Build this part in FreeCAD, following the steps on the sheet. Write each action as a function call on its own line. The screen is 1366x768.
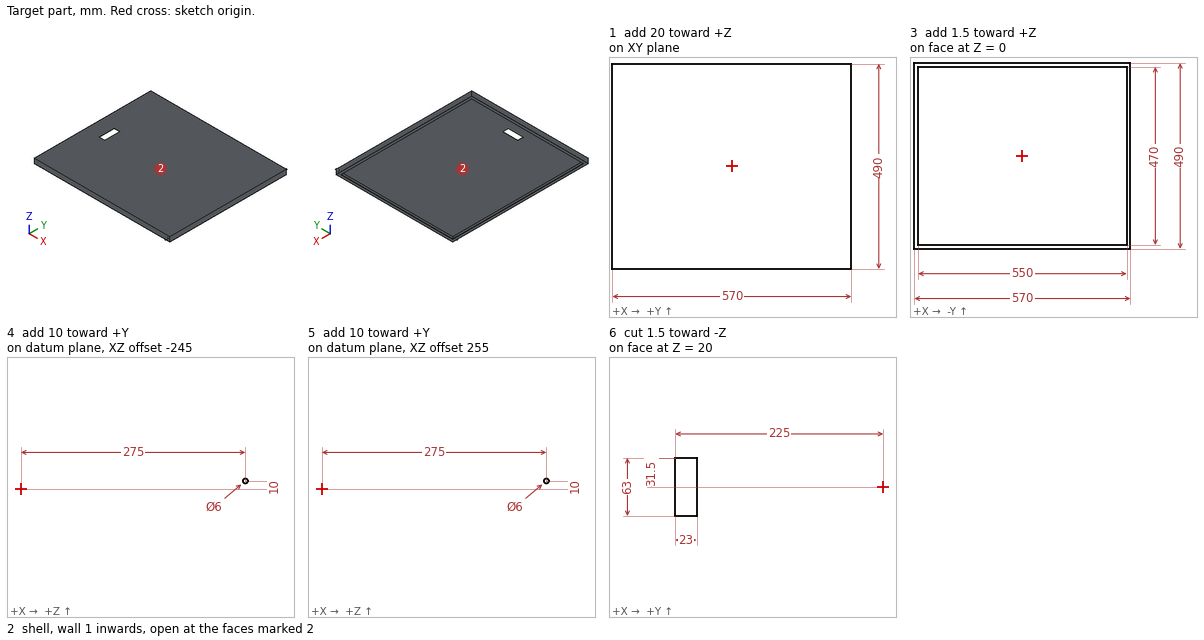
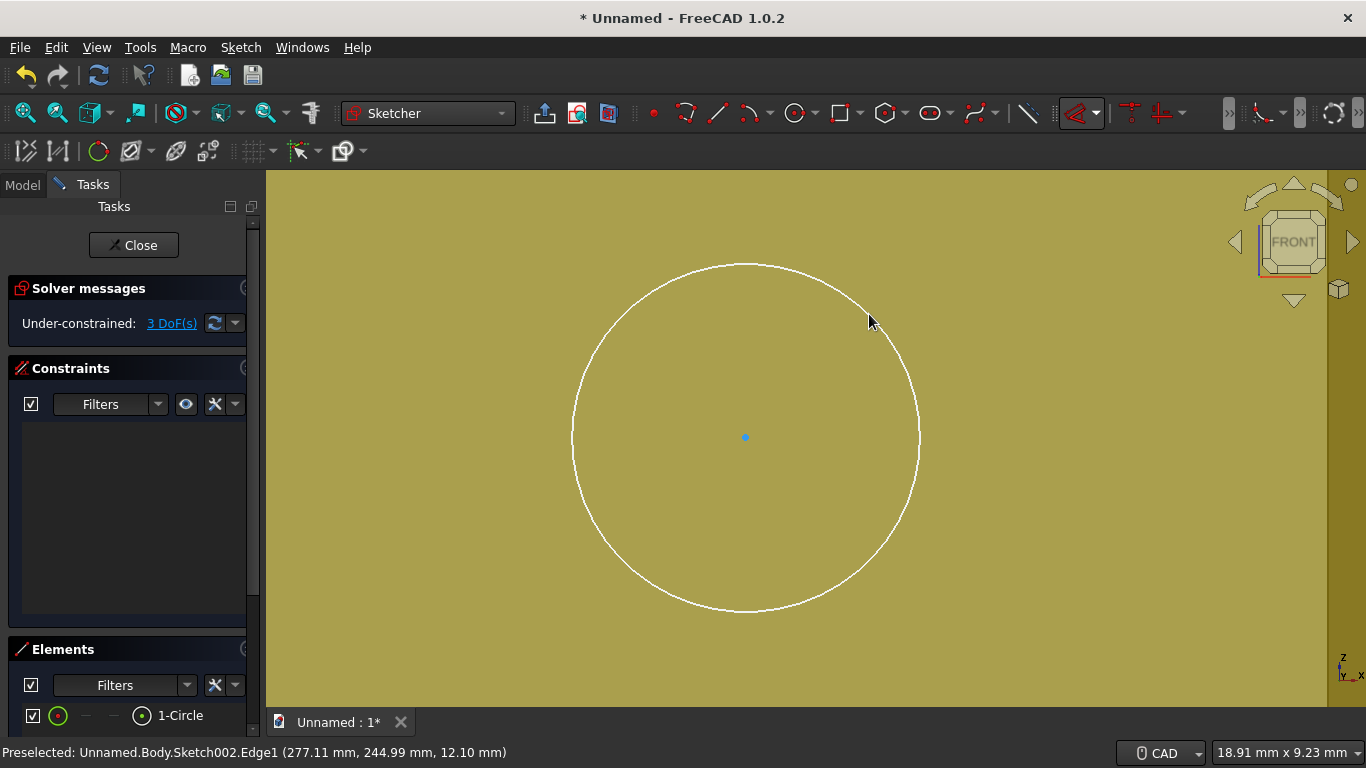
click(869, 315)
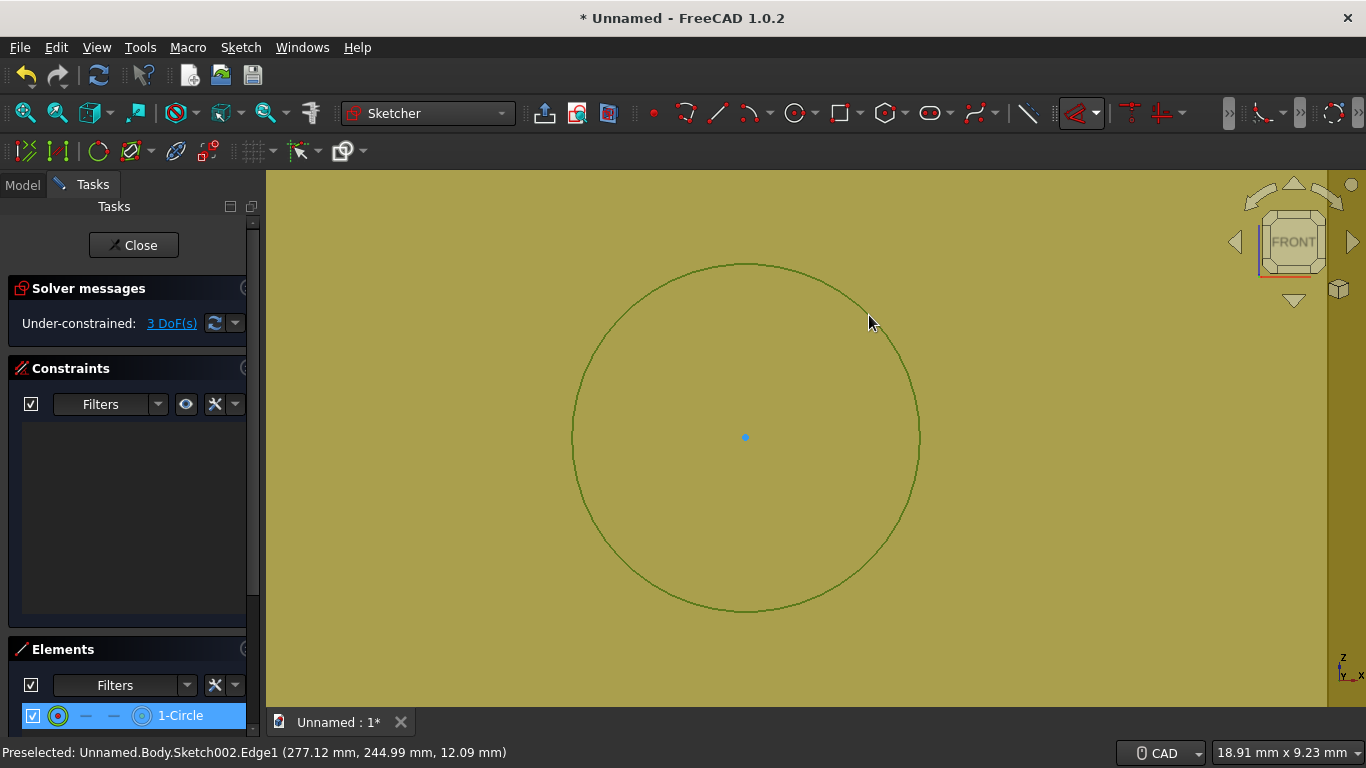
key(k)
key(o)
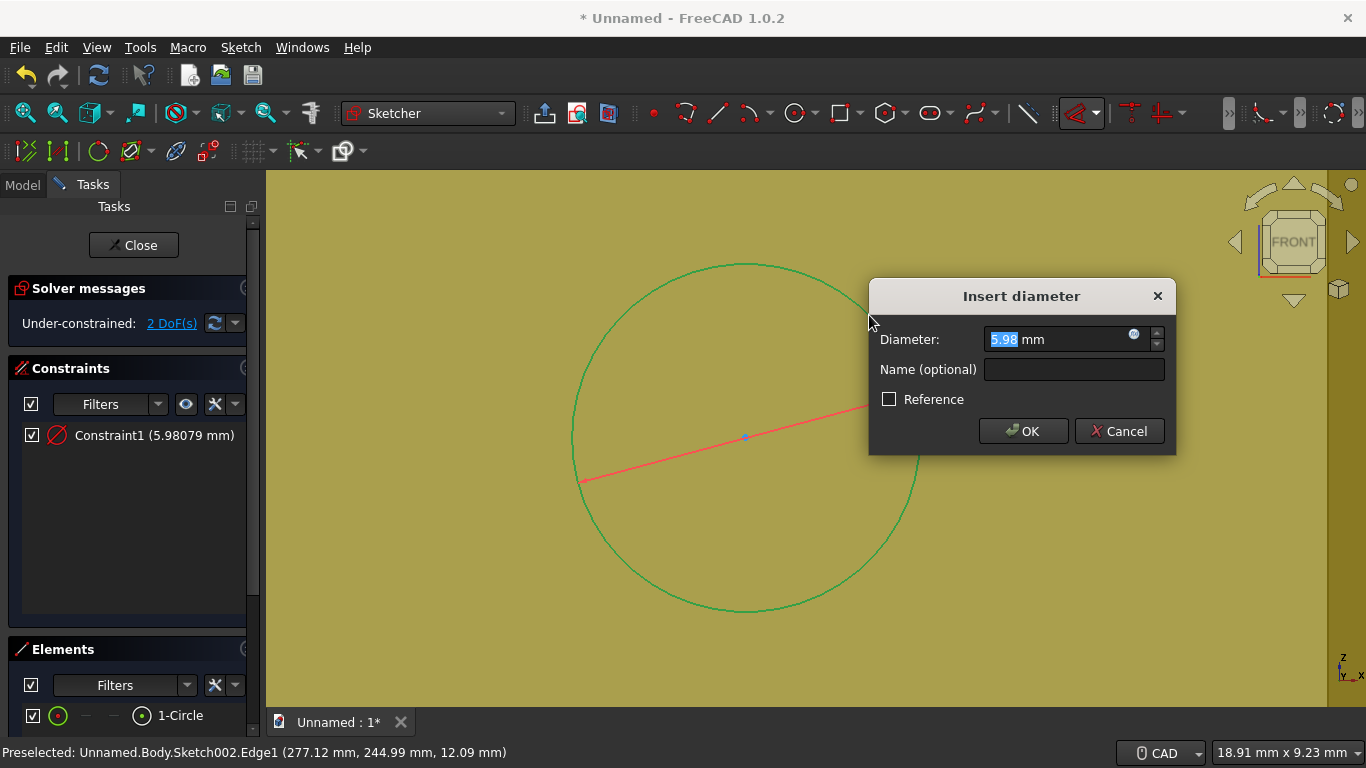
text(6)
key(Return)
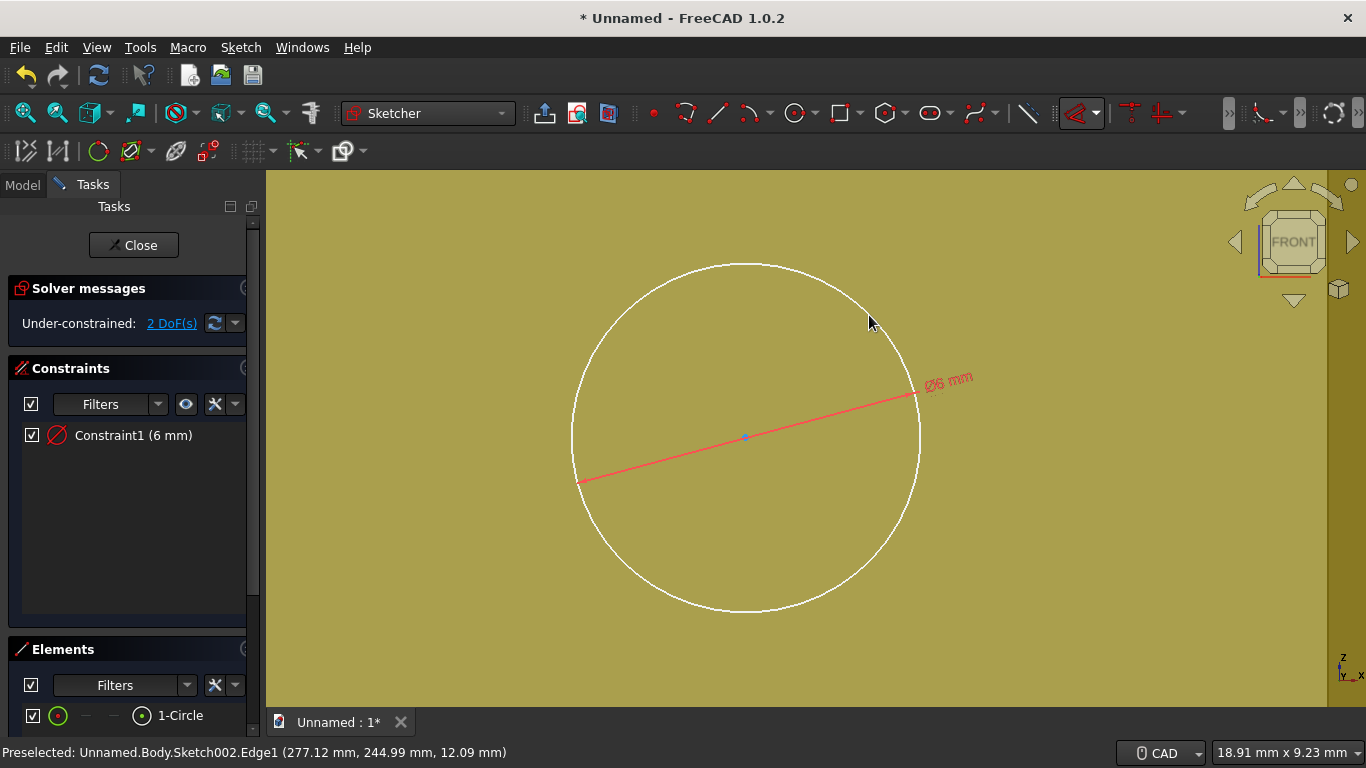
click(746, 438)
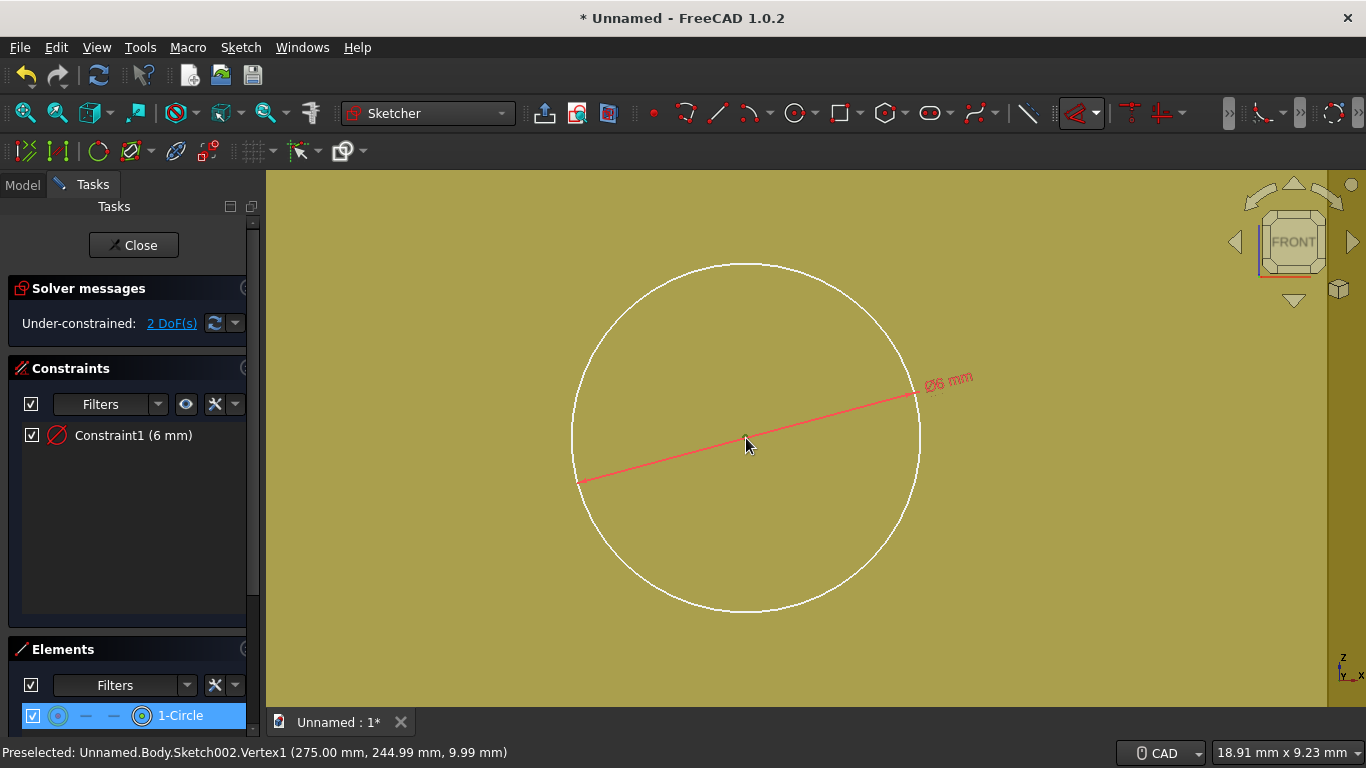
key(i)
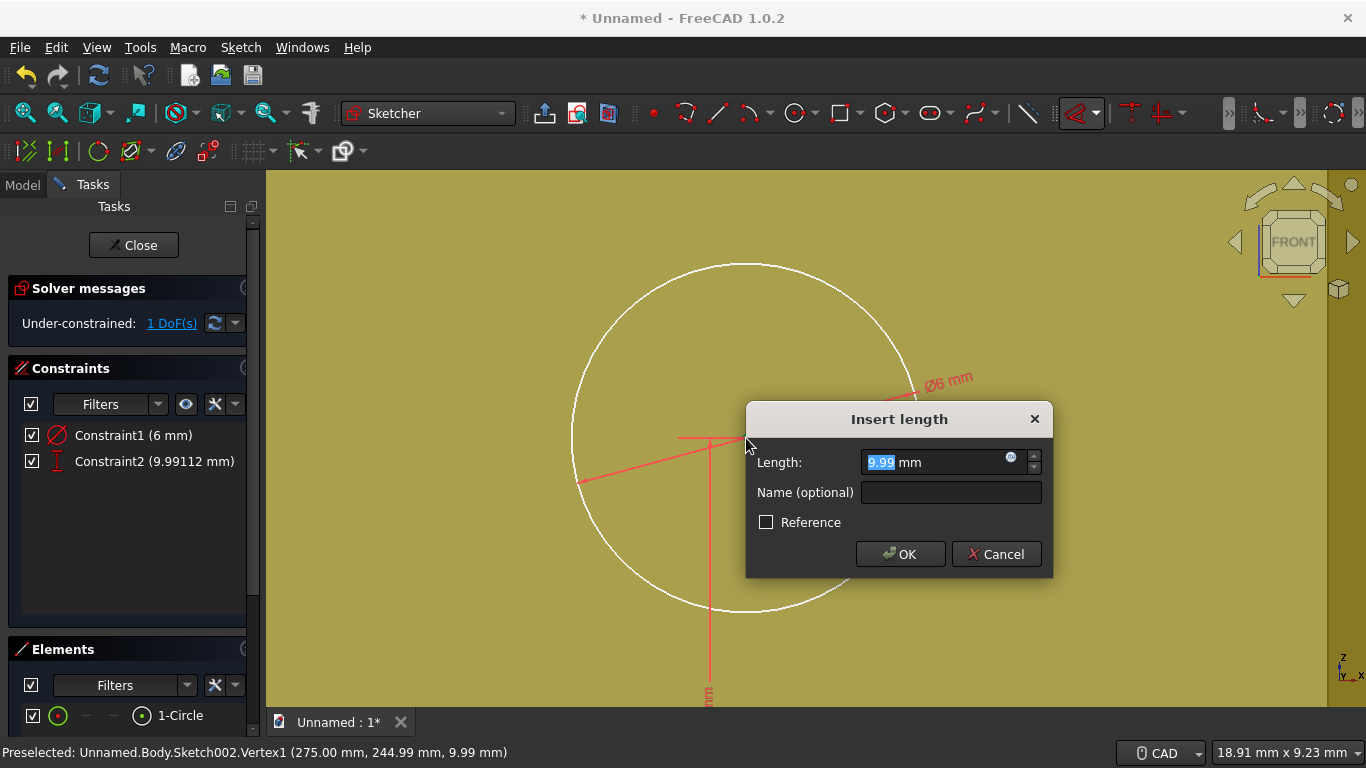
text(10)
key(Return)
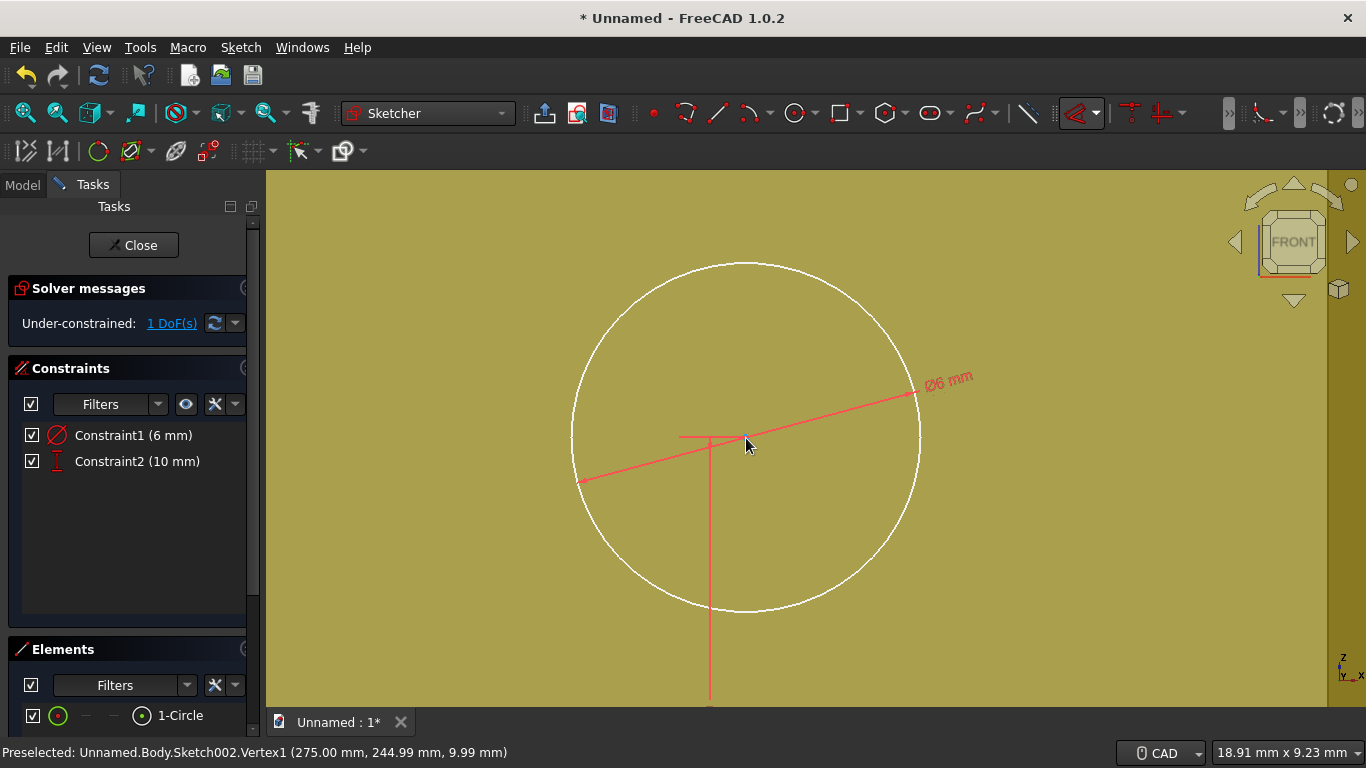
click(746, 437)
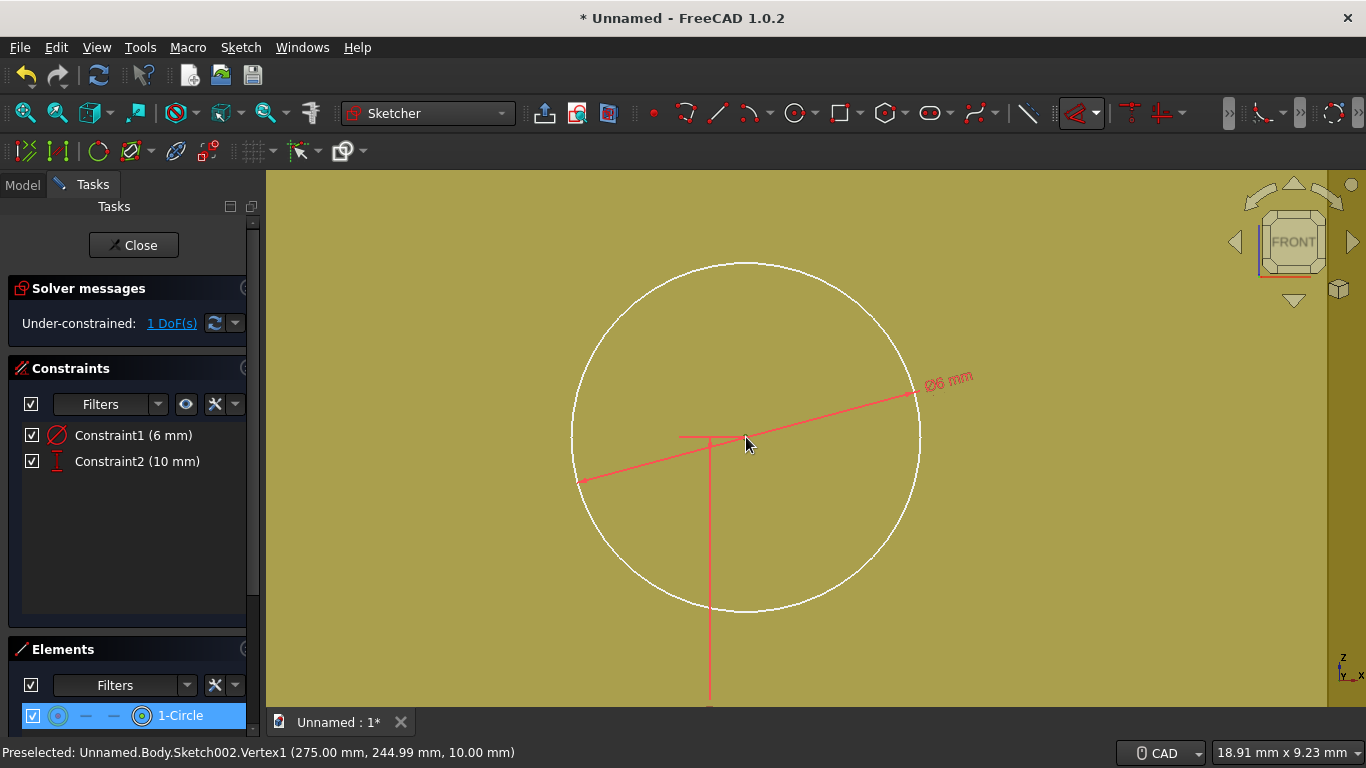
key(l)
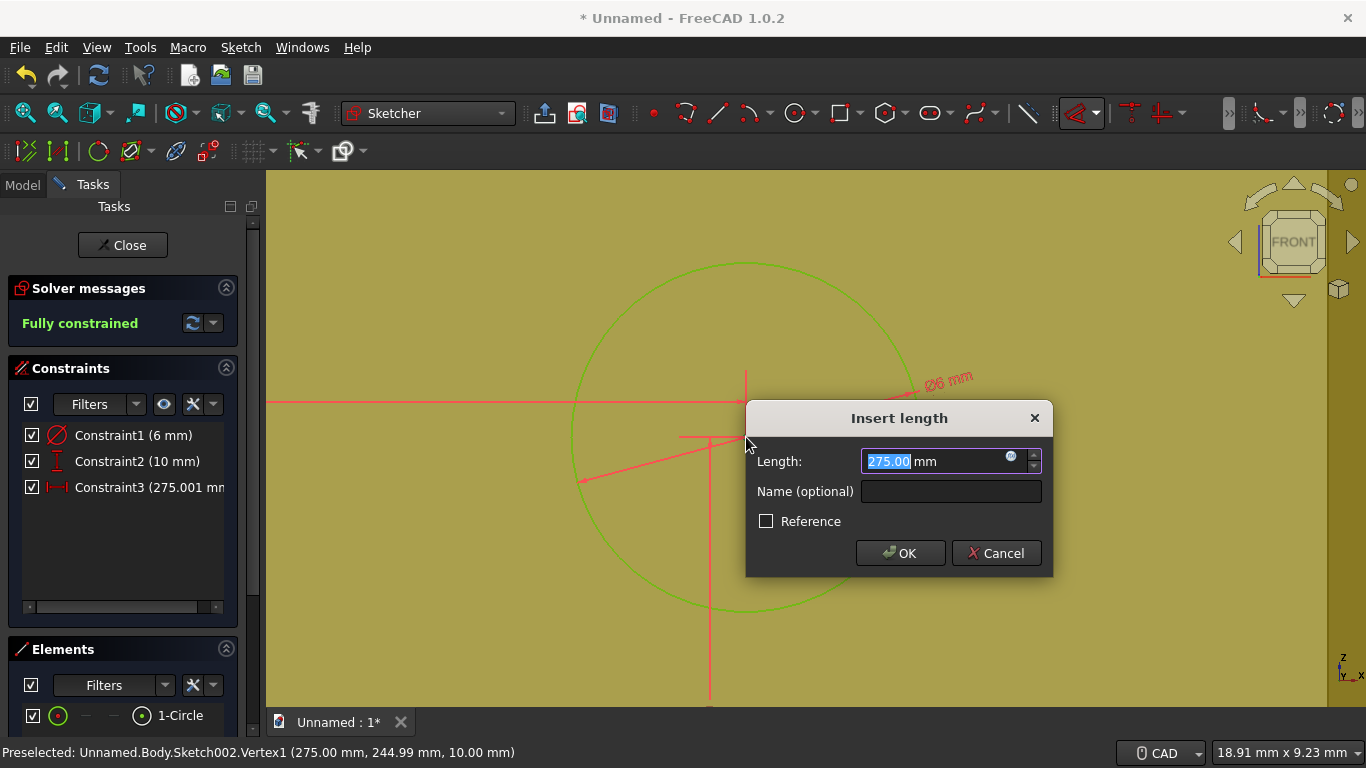
text(275)
key(Return)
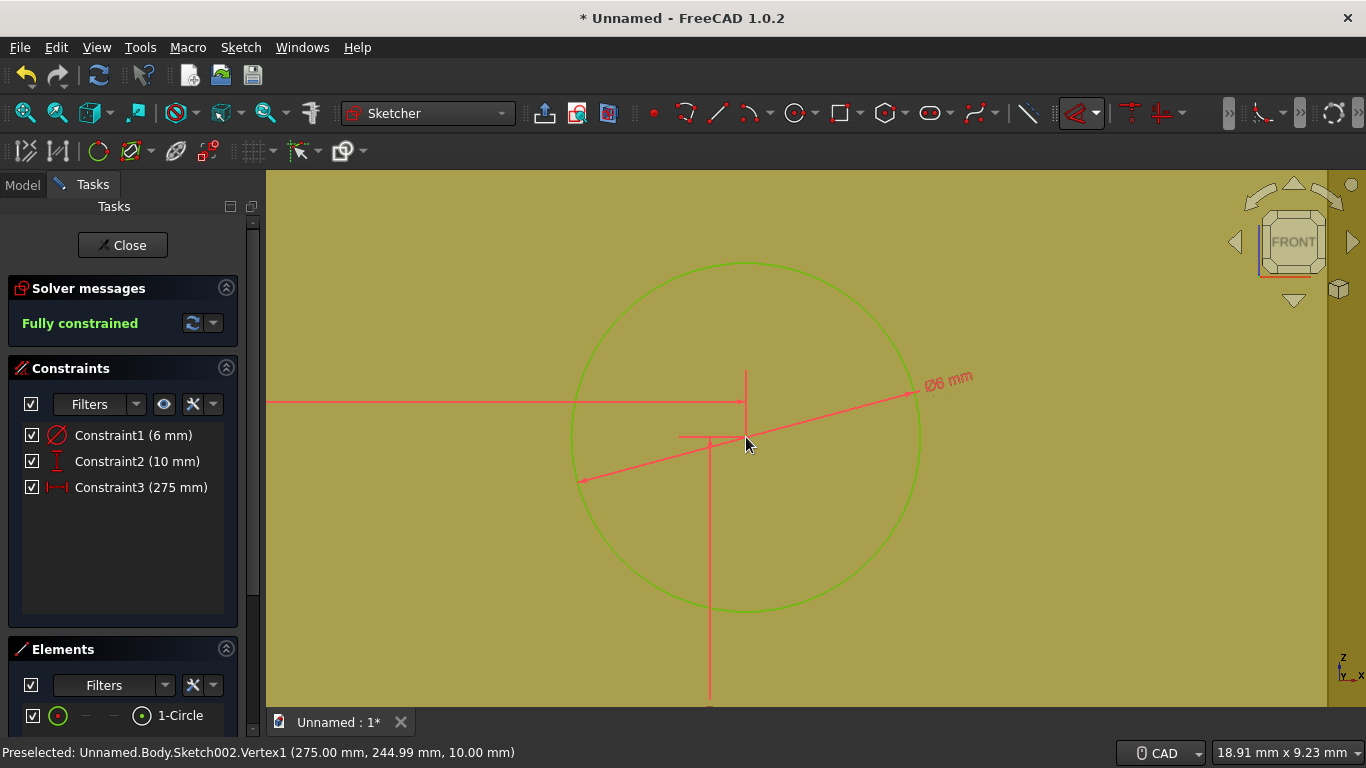
click(123, 245)